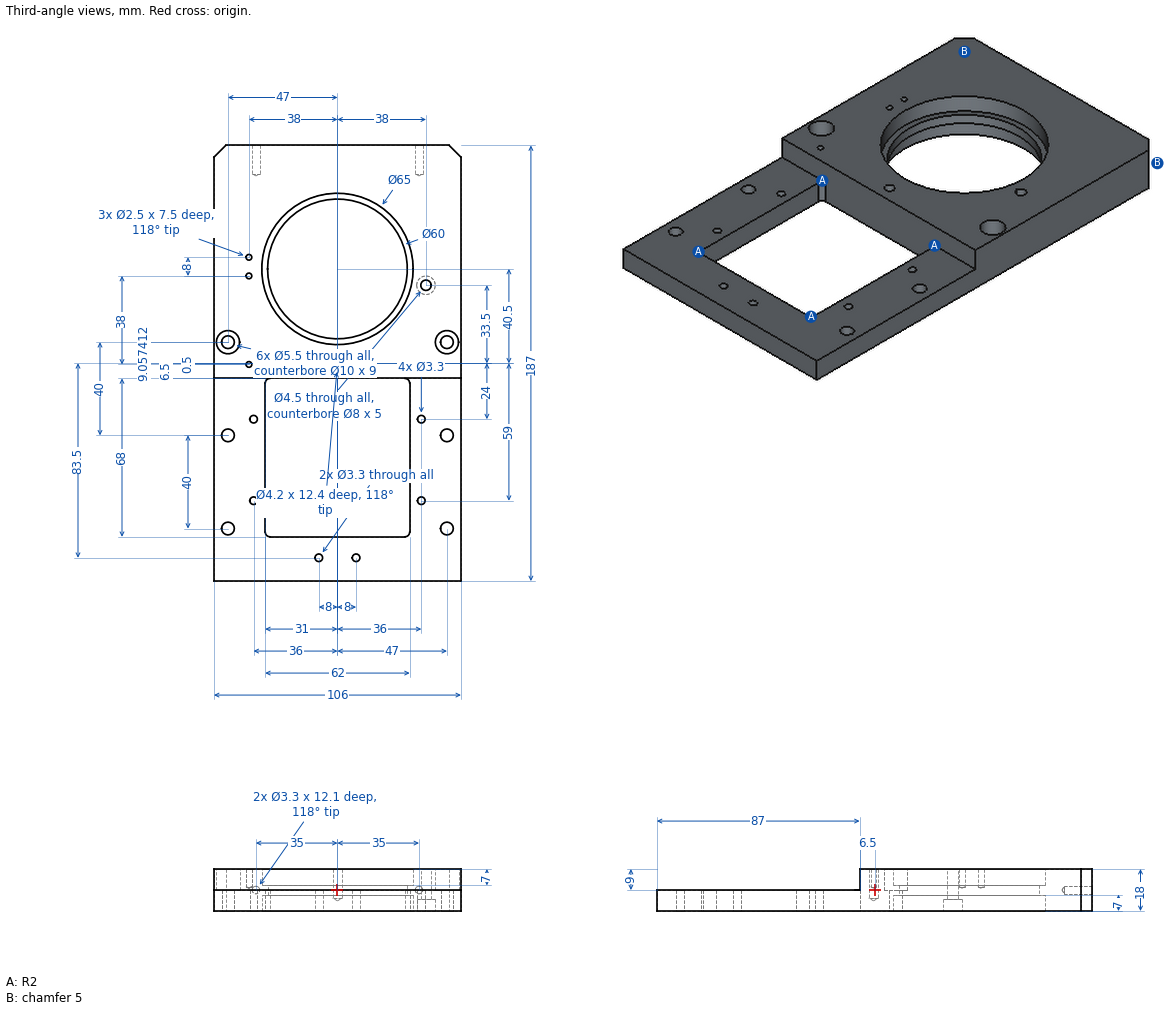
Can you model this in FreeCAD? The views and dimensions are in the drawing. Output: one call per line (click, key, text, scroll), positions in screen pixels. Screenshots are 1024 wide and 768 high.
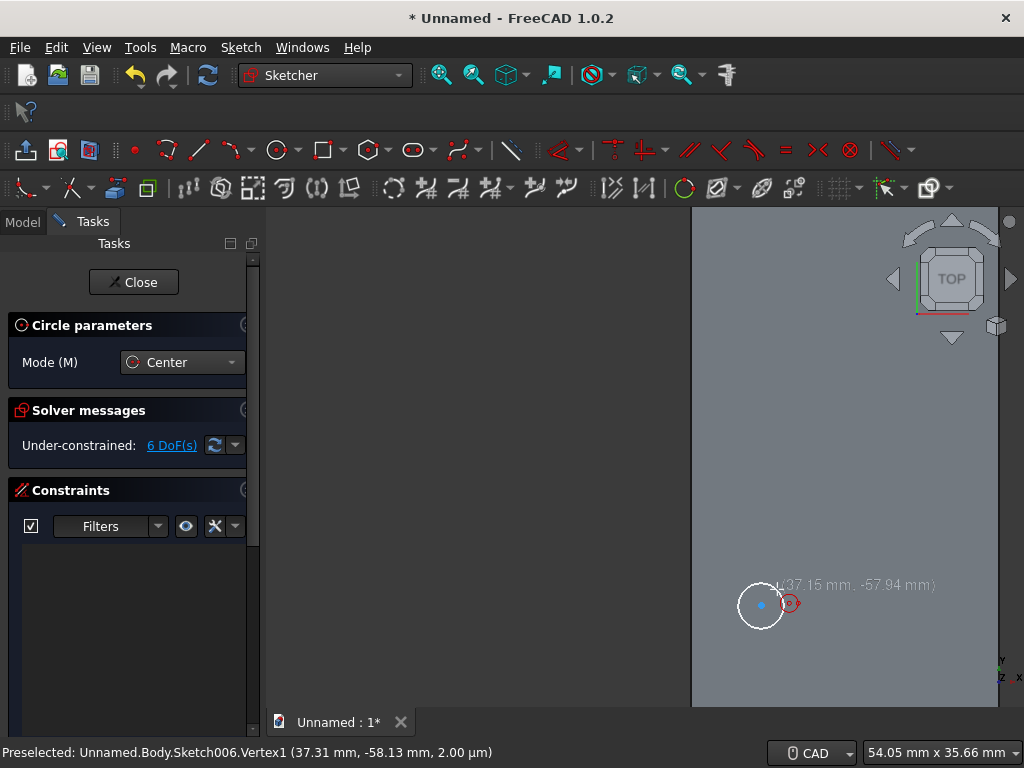
scroll(763, 605, down, 5)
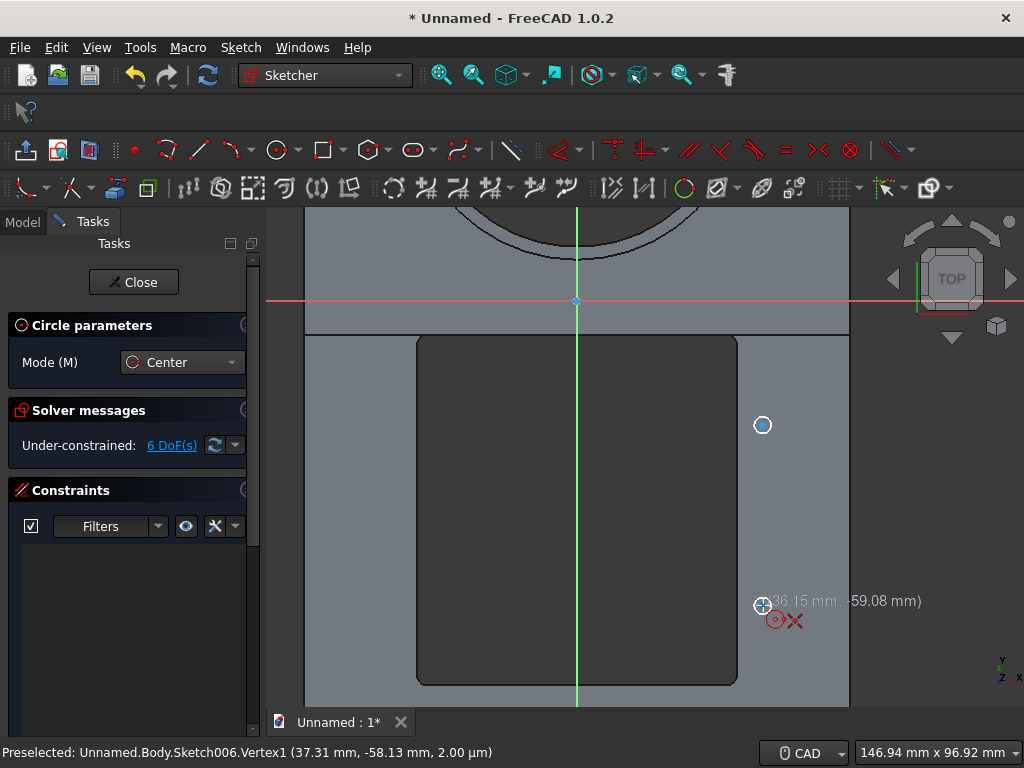
scroll(391, 605, up, 5)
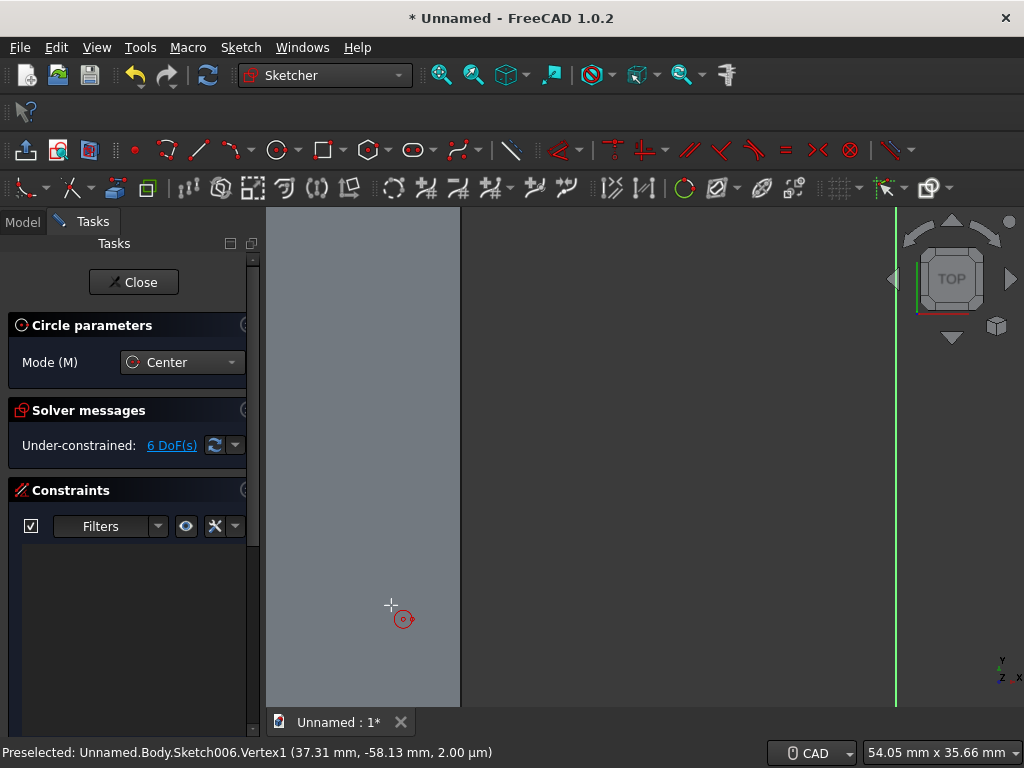
click(391, 605)
click(408, 589)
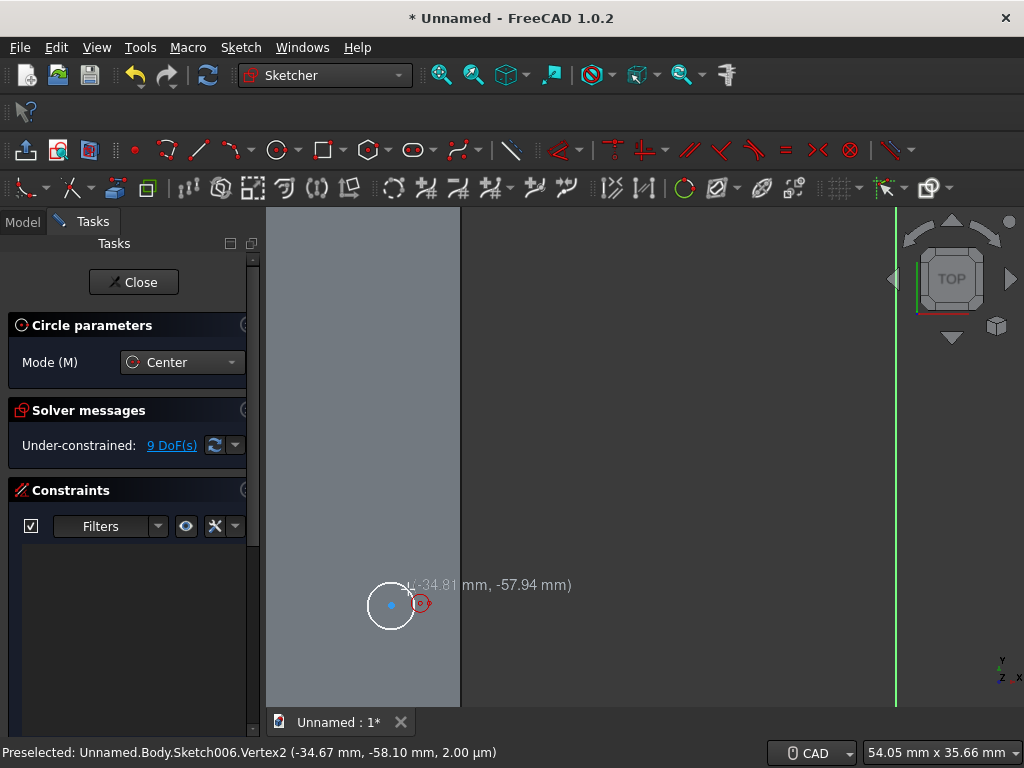
scroll(390, 605, down, 5)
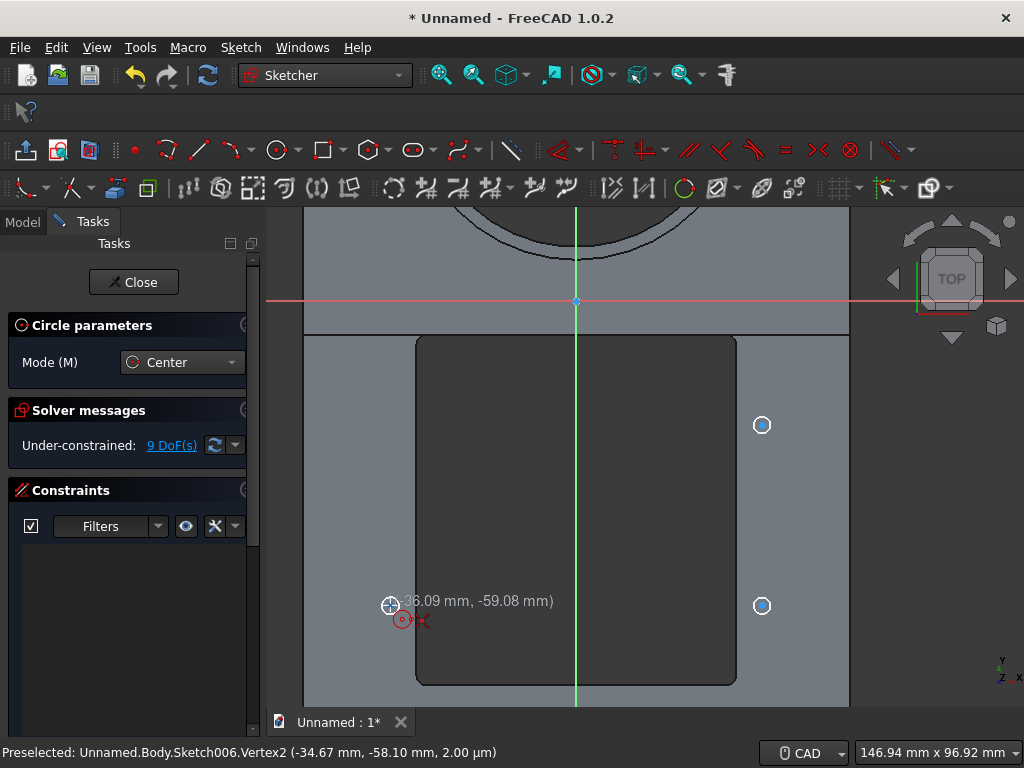
scroll(391, 425, up, 5)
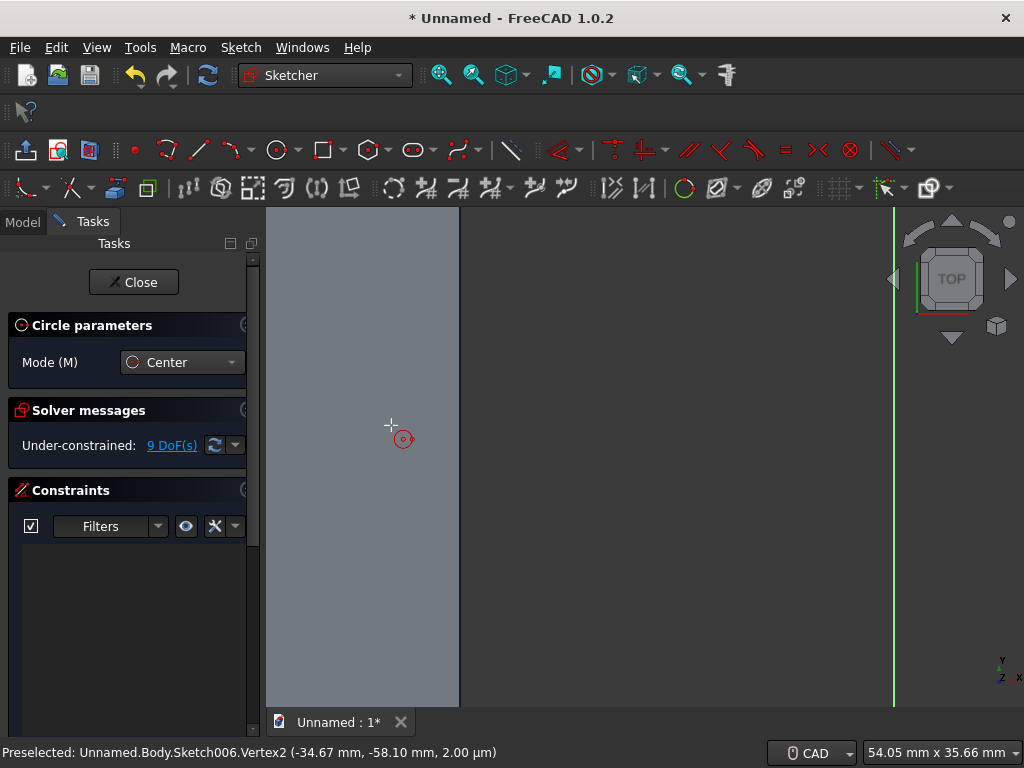
click(390, 424)
click(406, 408)
key(Escape)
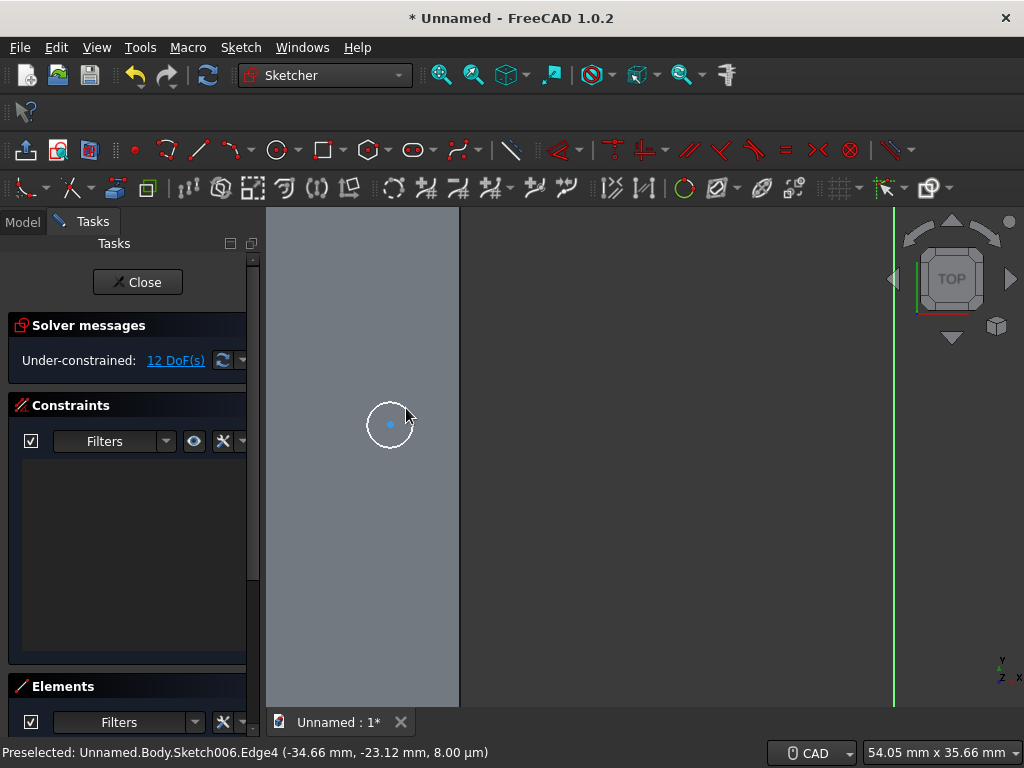
scroll(391, 425, down, 5)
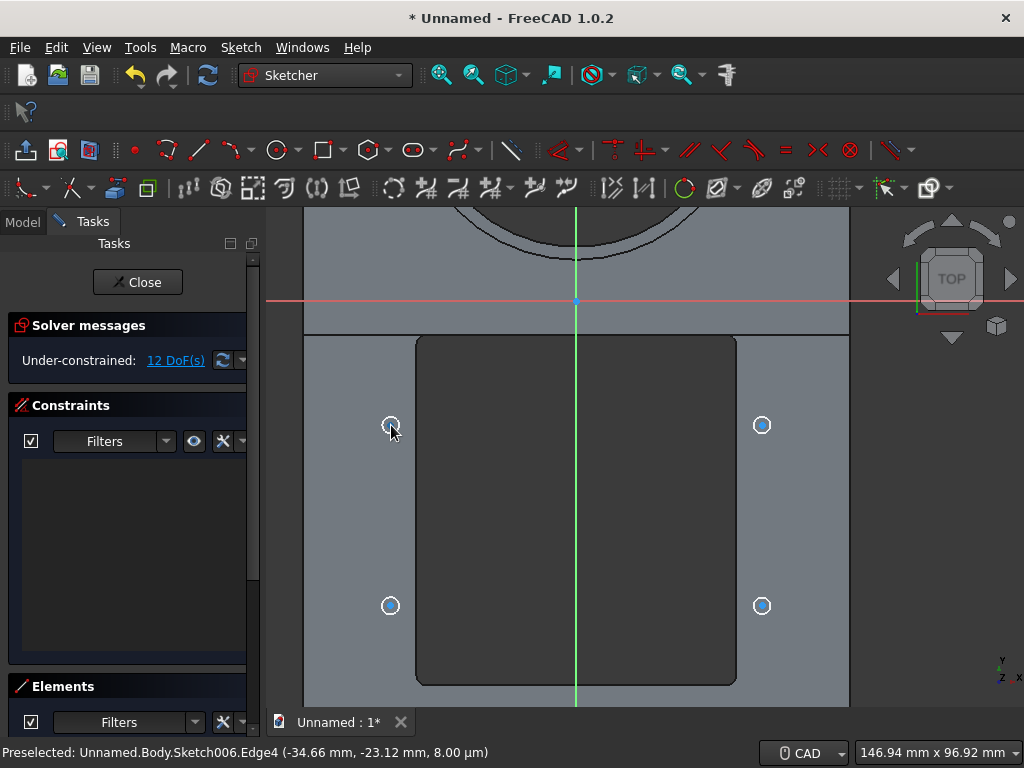
scroll(768, 419, up, 3)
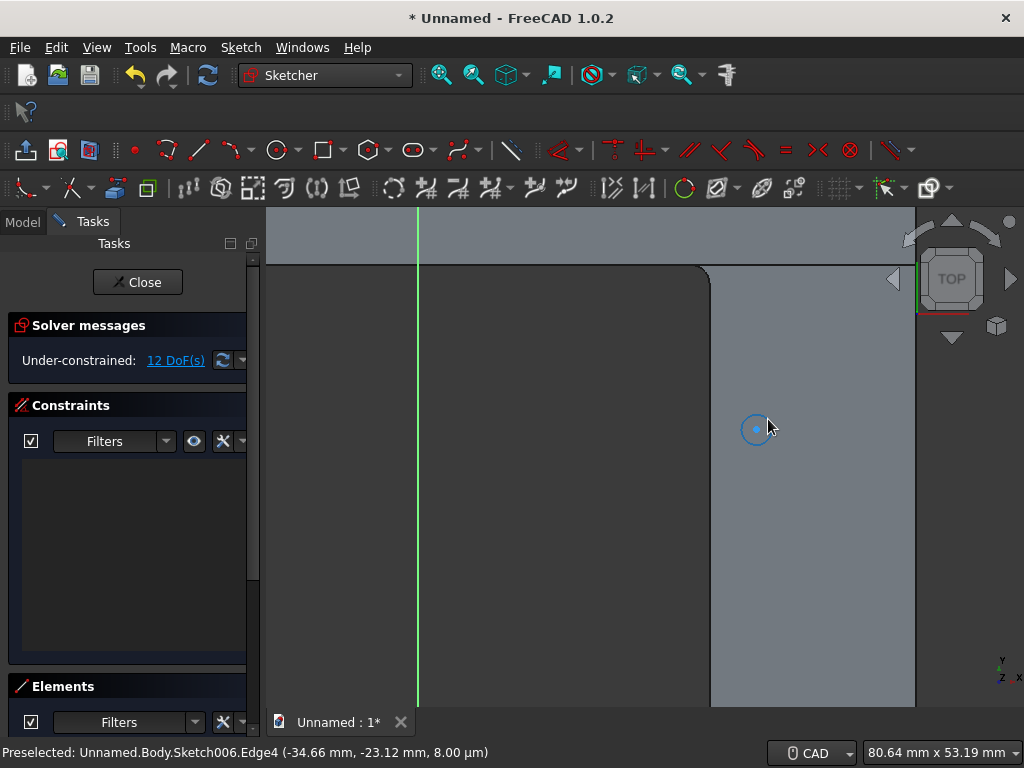
click(767, 419)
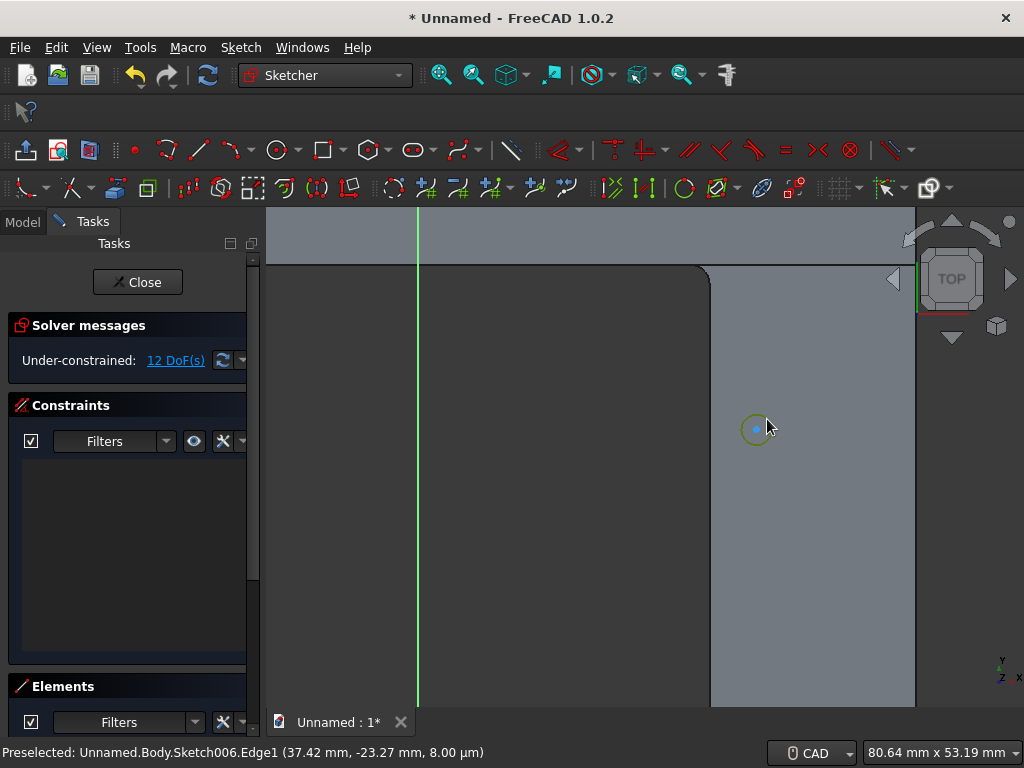
scroll(769, 418, down, 3)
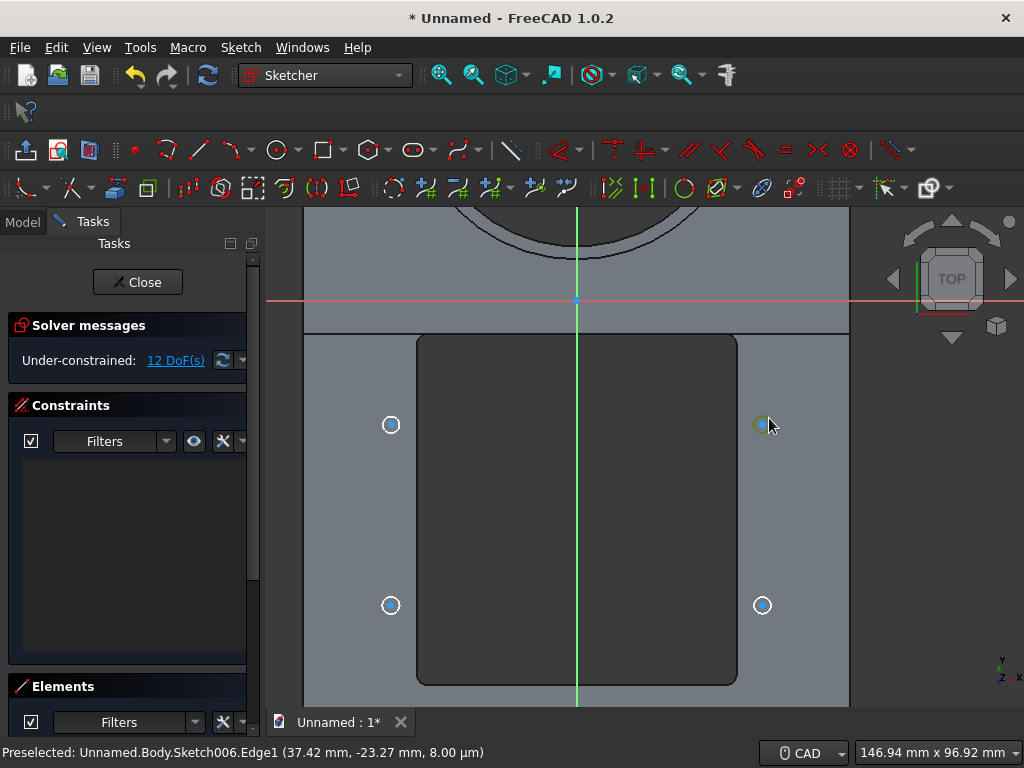
scroll(768, 600, up, 3)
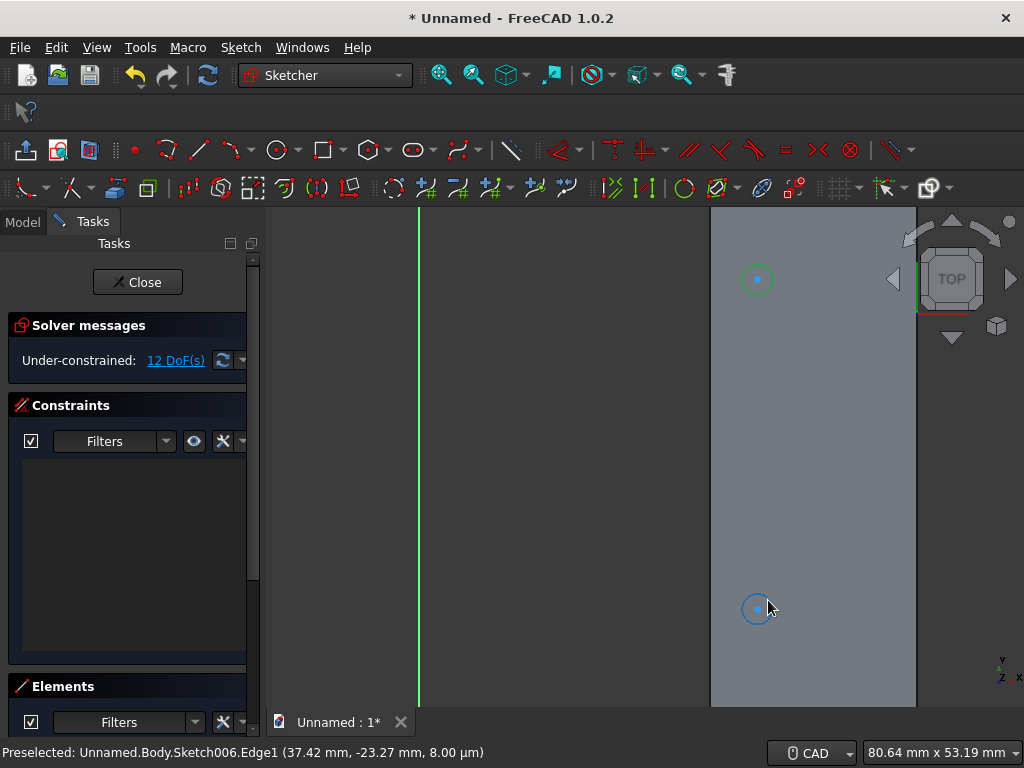
click(768, 598)